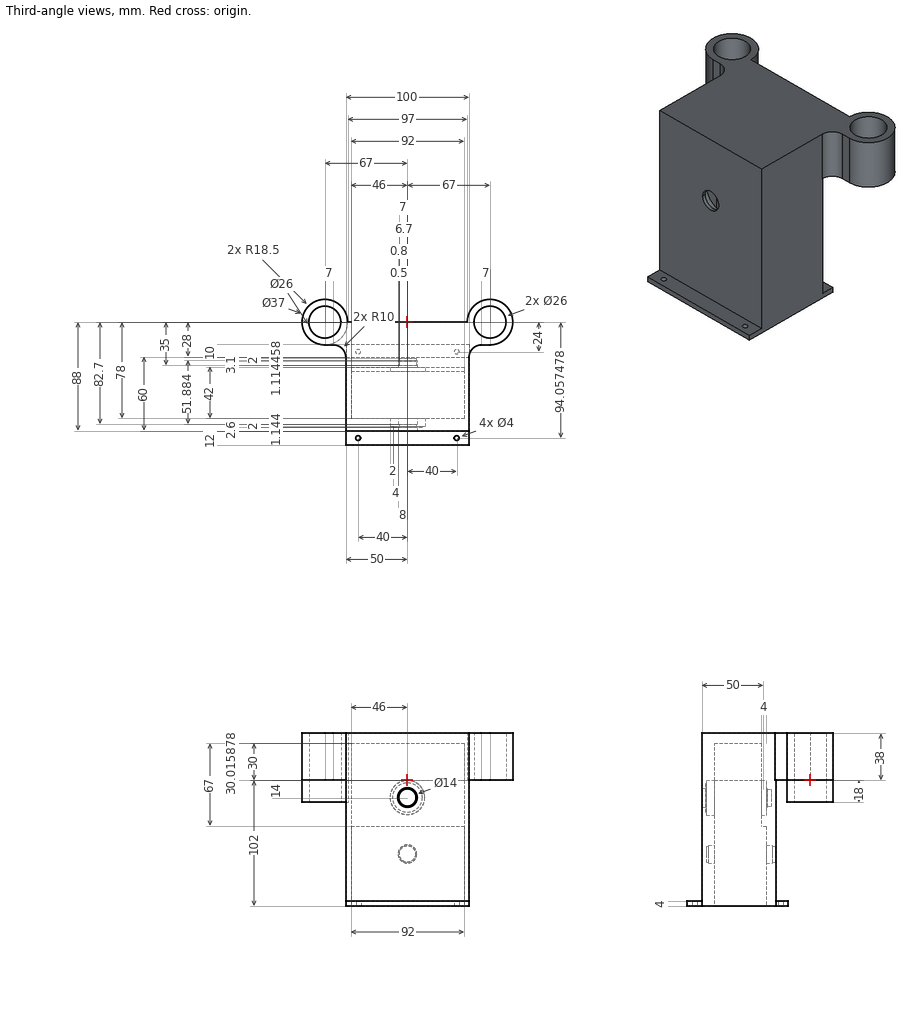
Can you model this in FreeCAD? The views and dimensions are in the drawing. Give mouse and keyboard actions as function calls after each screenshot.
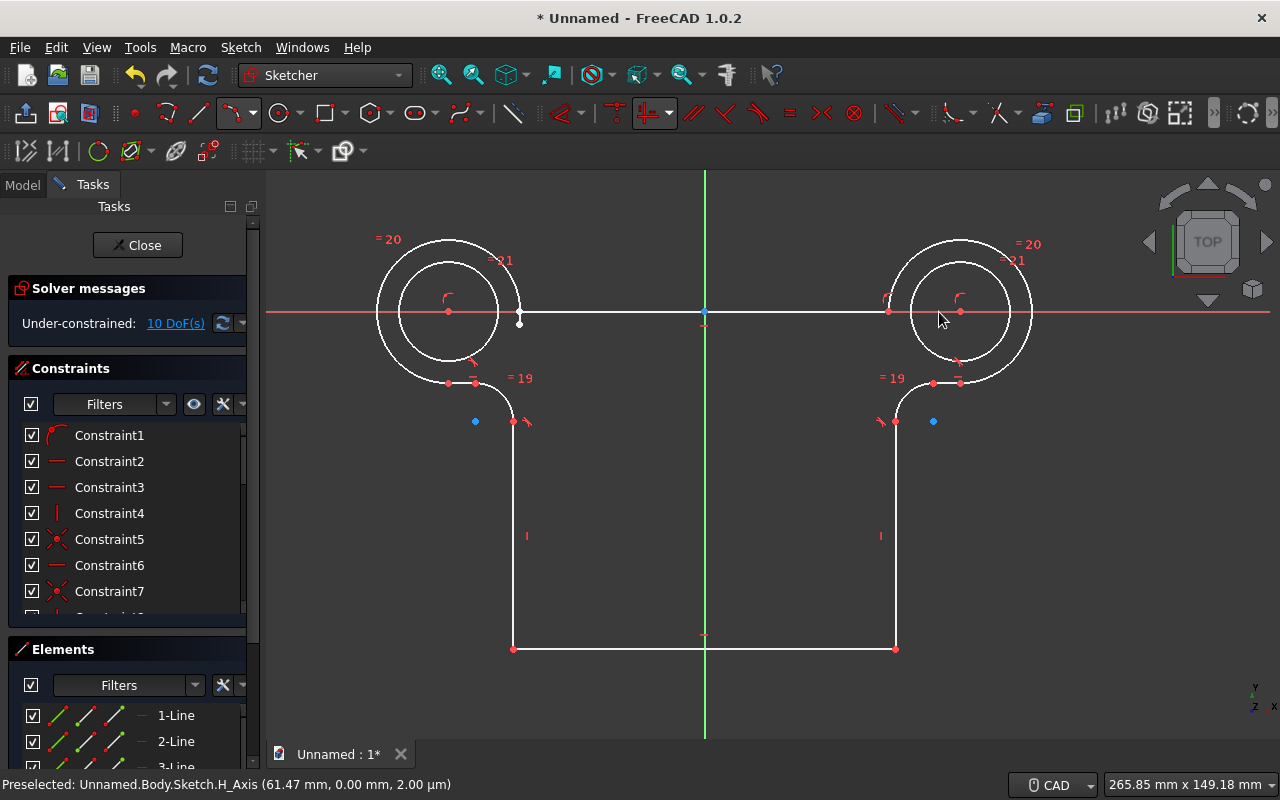
key(d)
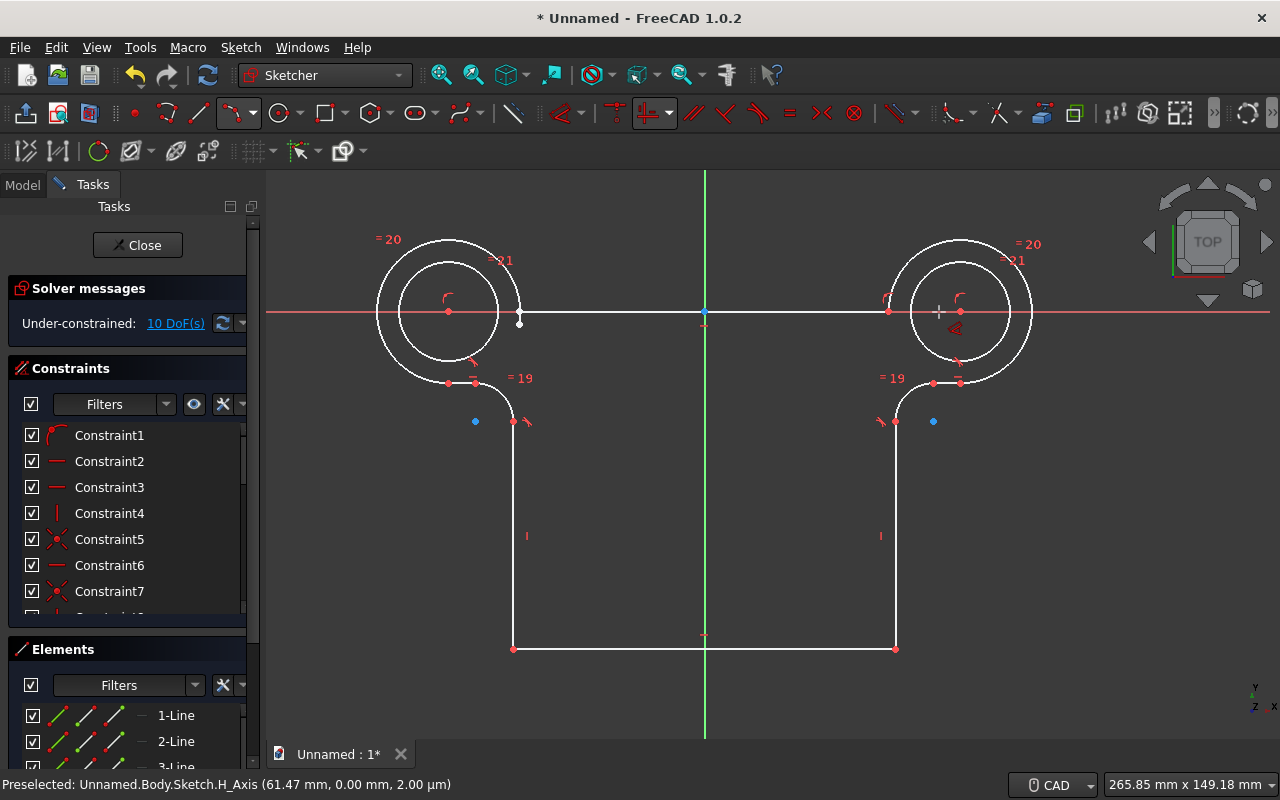
click(468, 243)
click(477, 212)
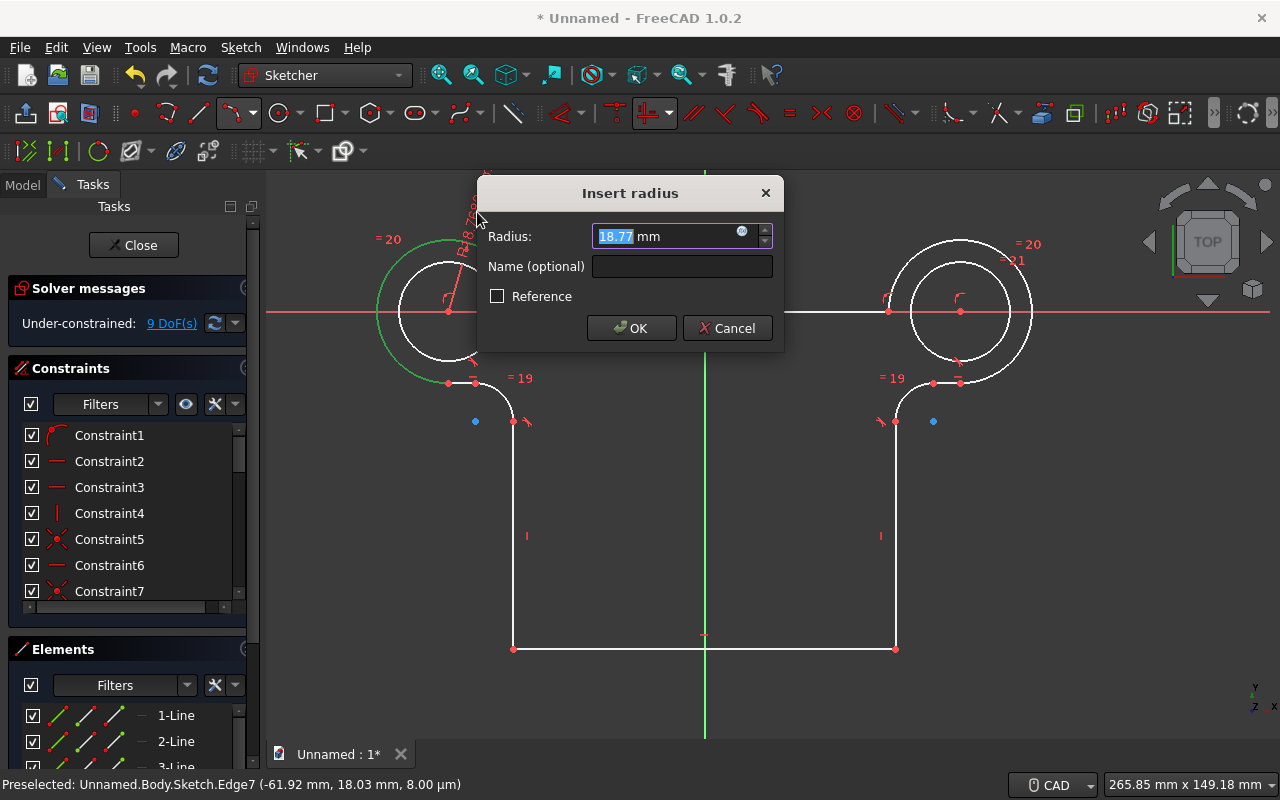
text(18.5)
key(Return)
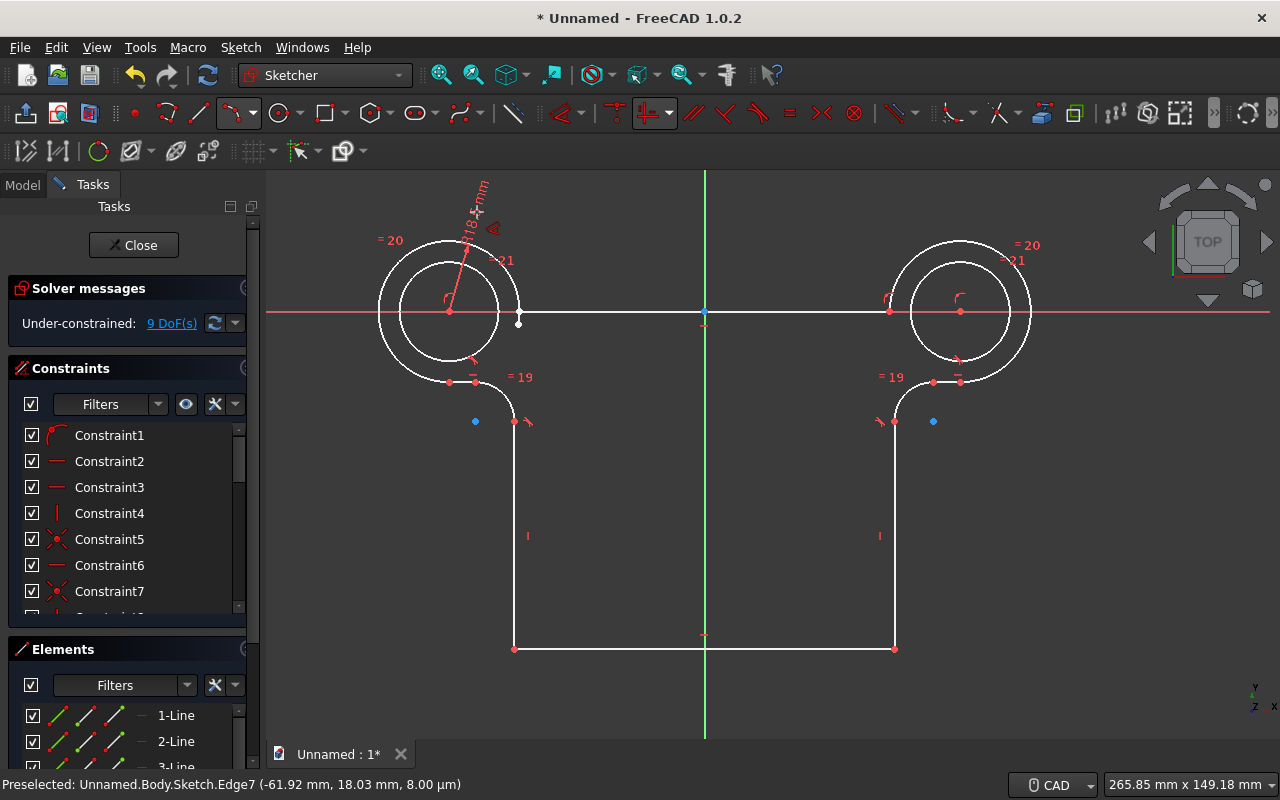
click(510, 403)
click(538, 388)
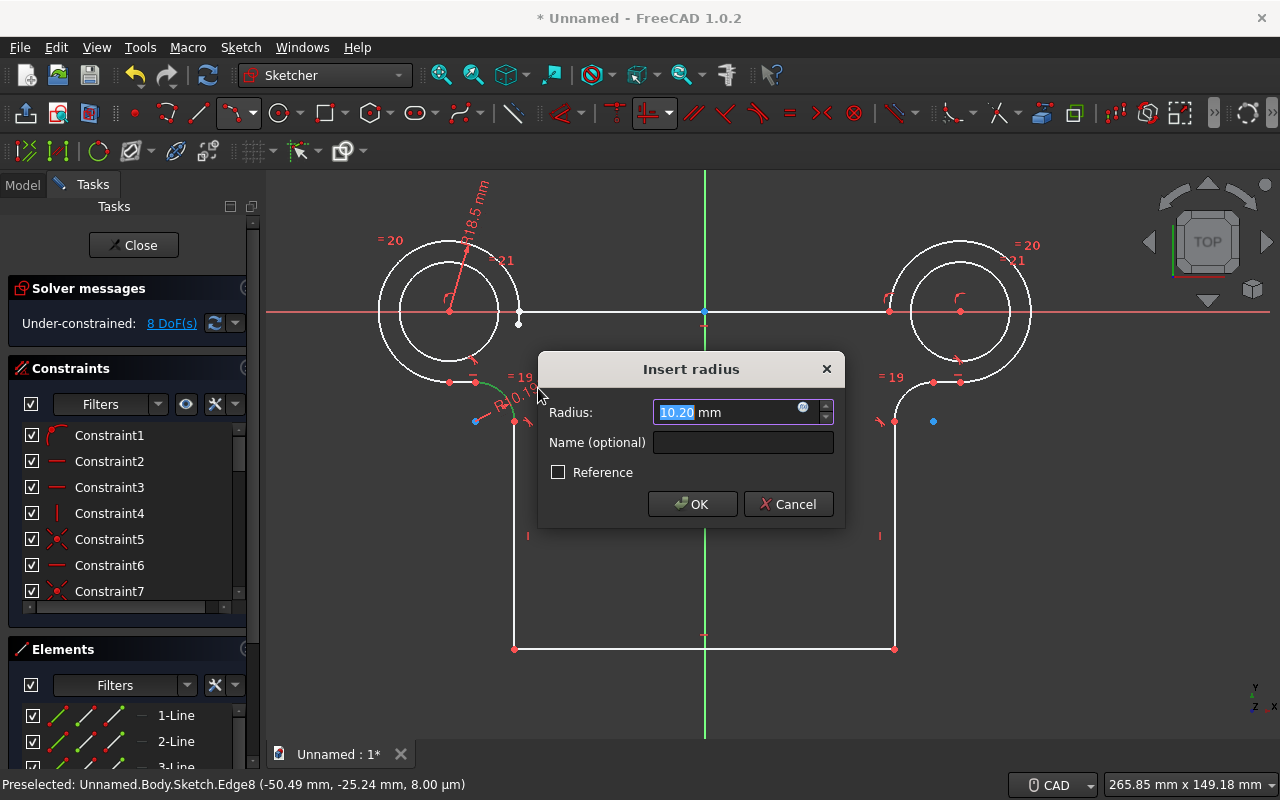
text(10)
key(Return)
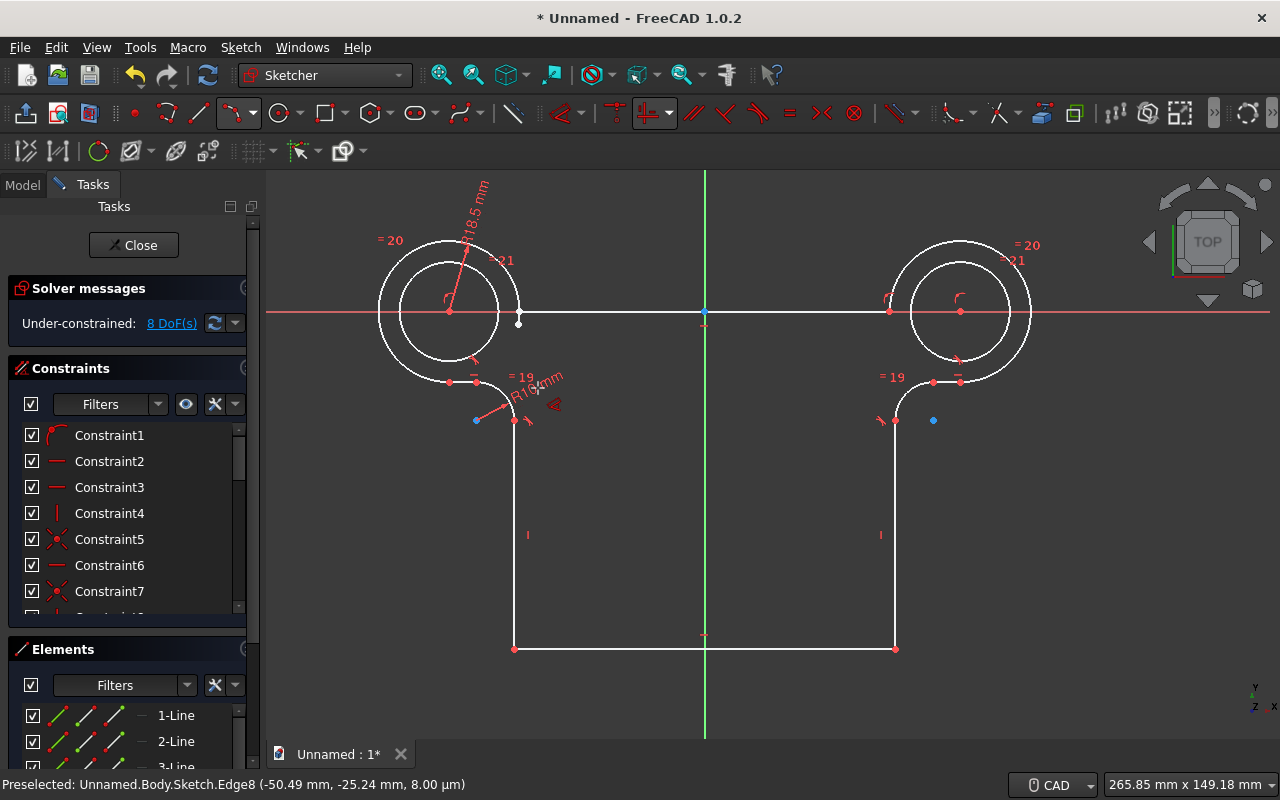
click(995, 277)
click(903, 369)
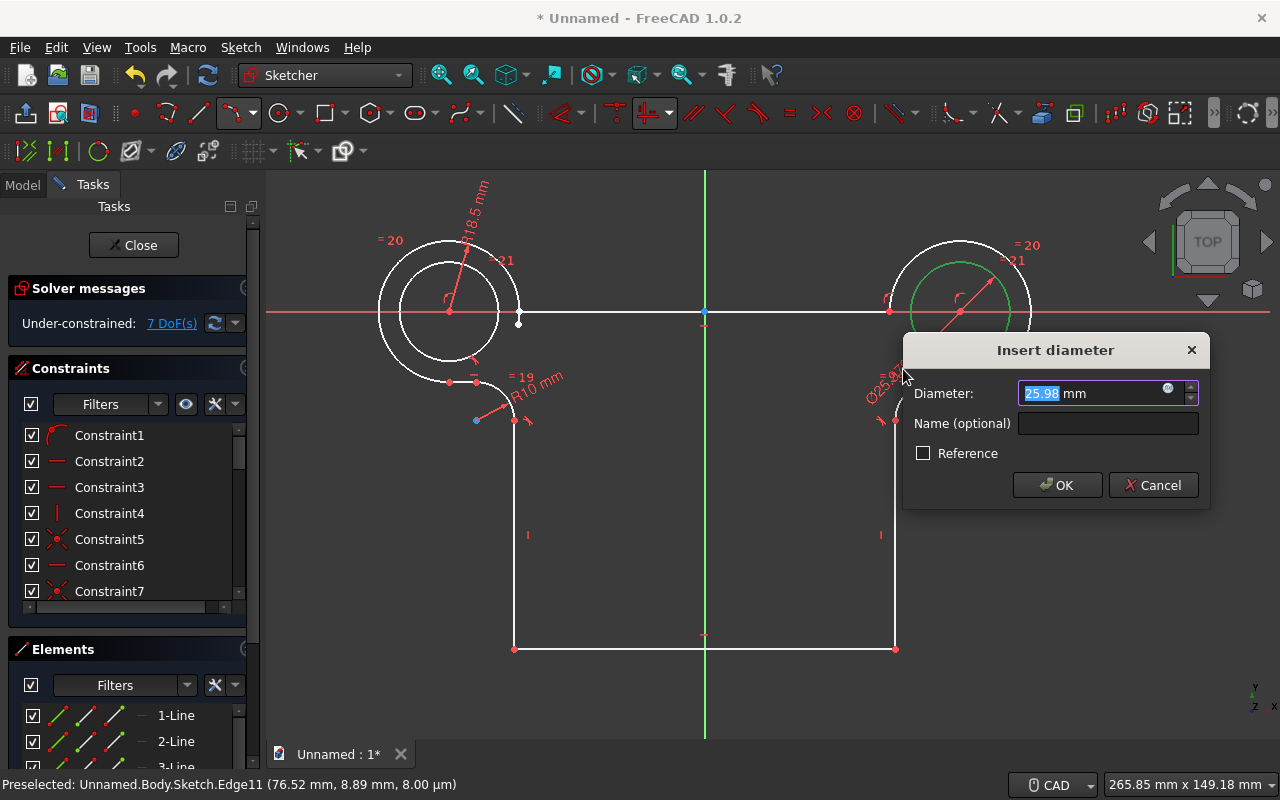
text(26)
key(Return)
key(Escape)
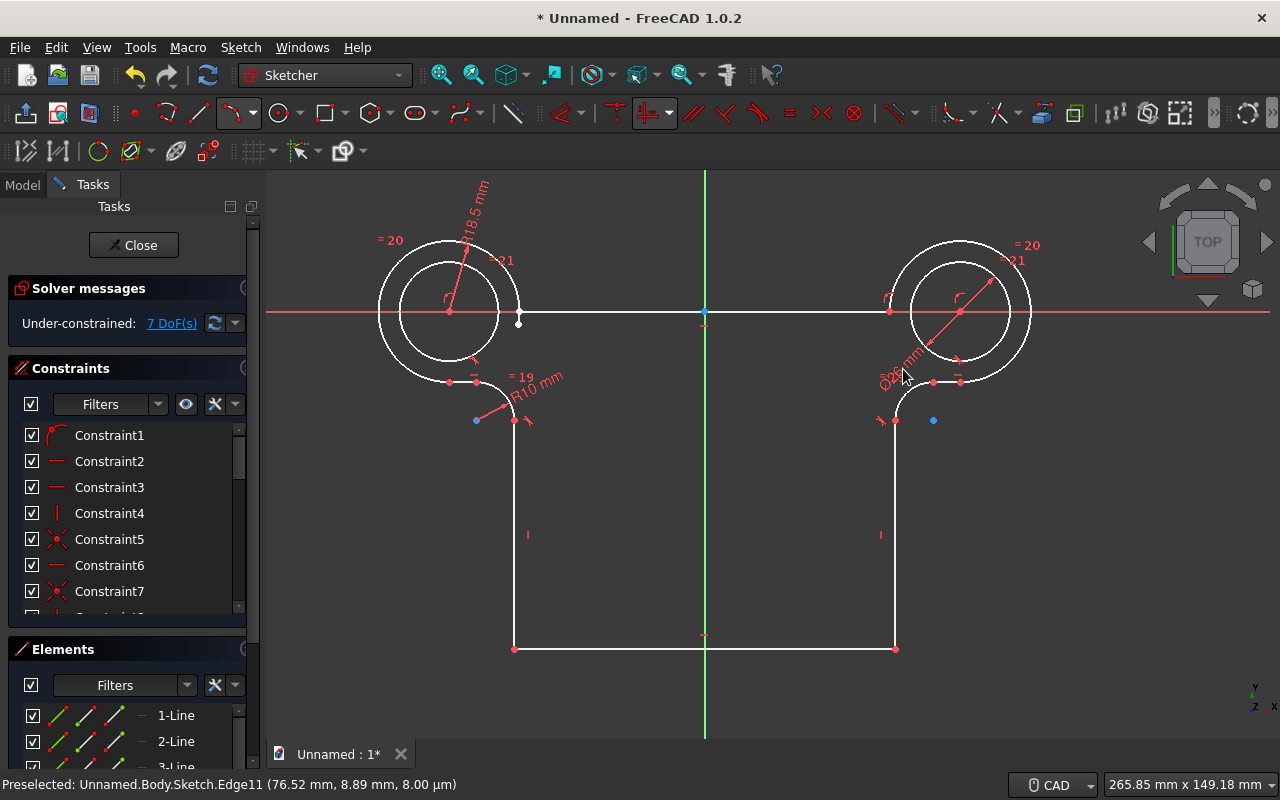
click(519, 324)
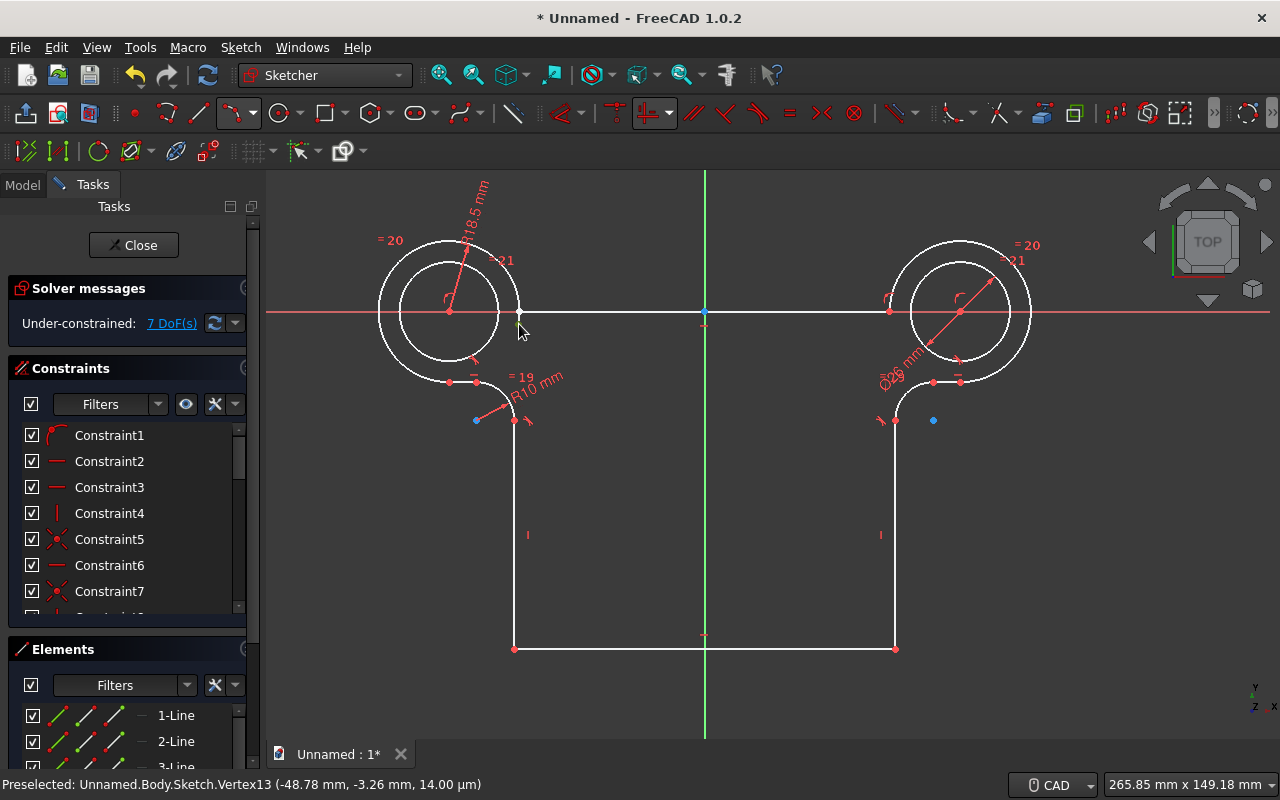
click(470, 312)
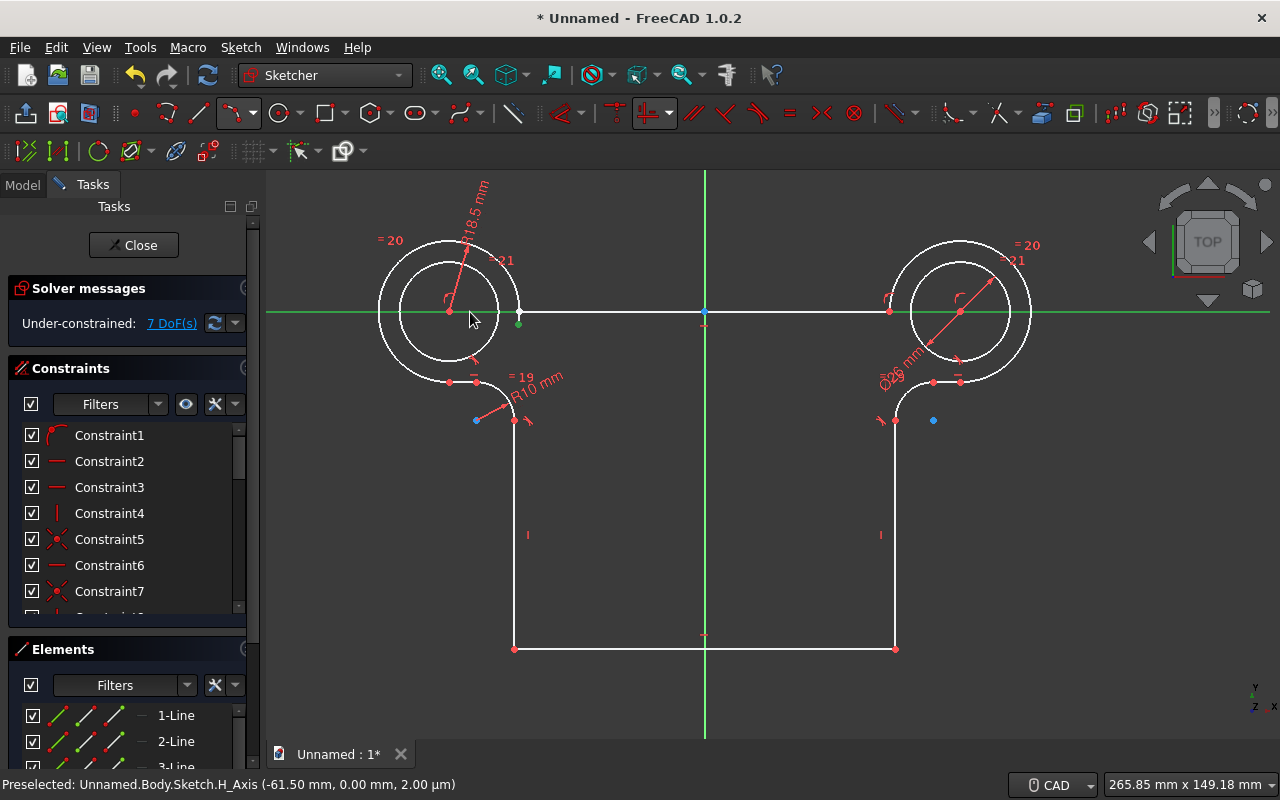
key(c)